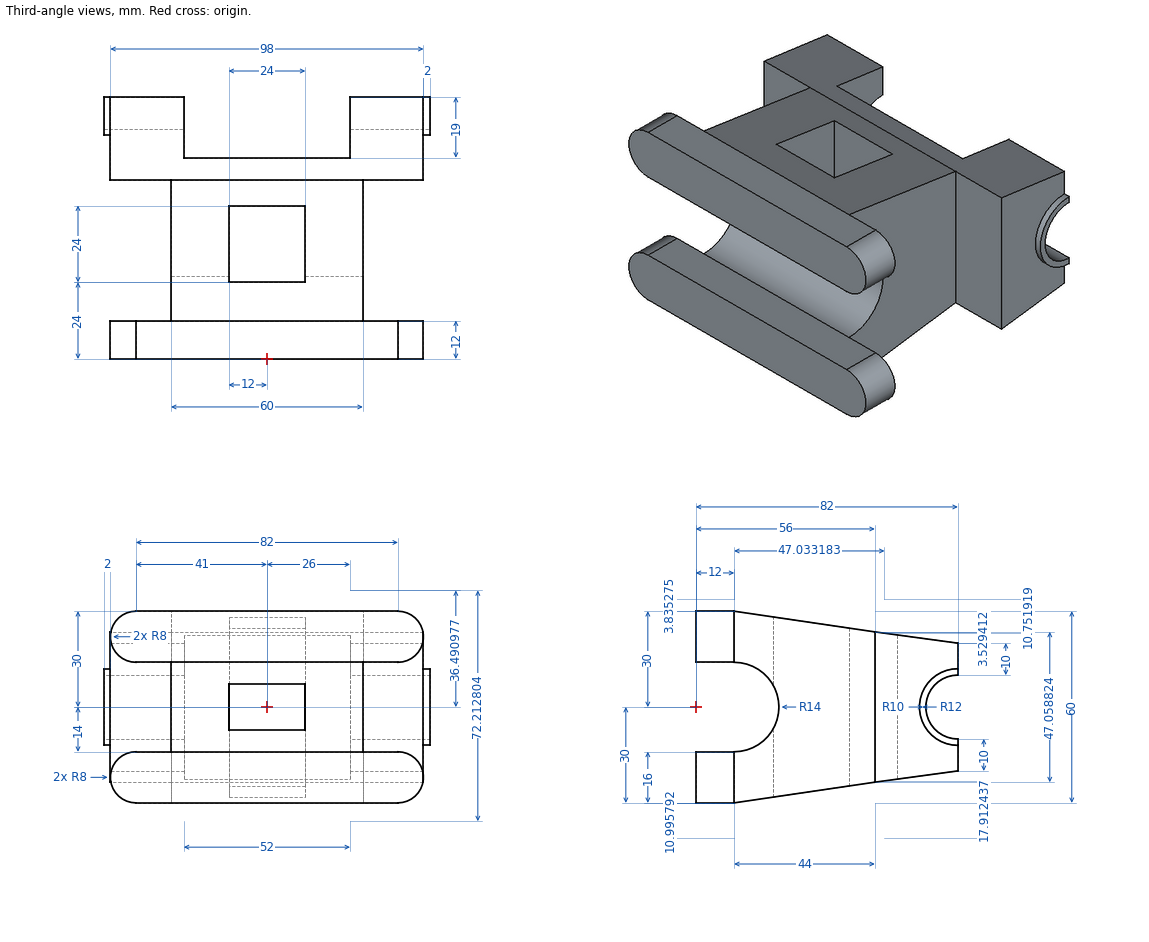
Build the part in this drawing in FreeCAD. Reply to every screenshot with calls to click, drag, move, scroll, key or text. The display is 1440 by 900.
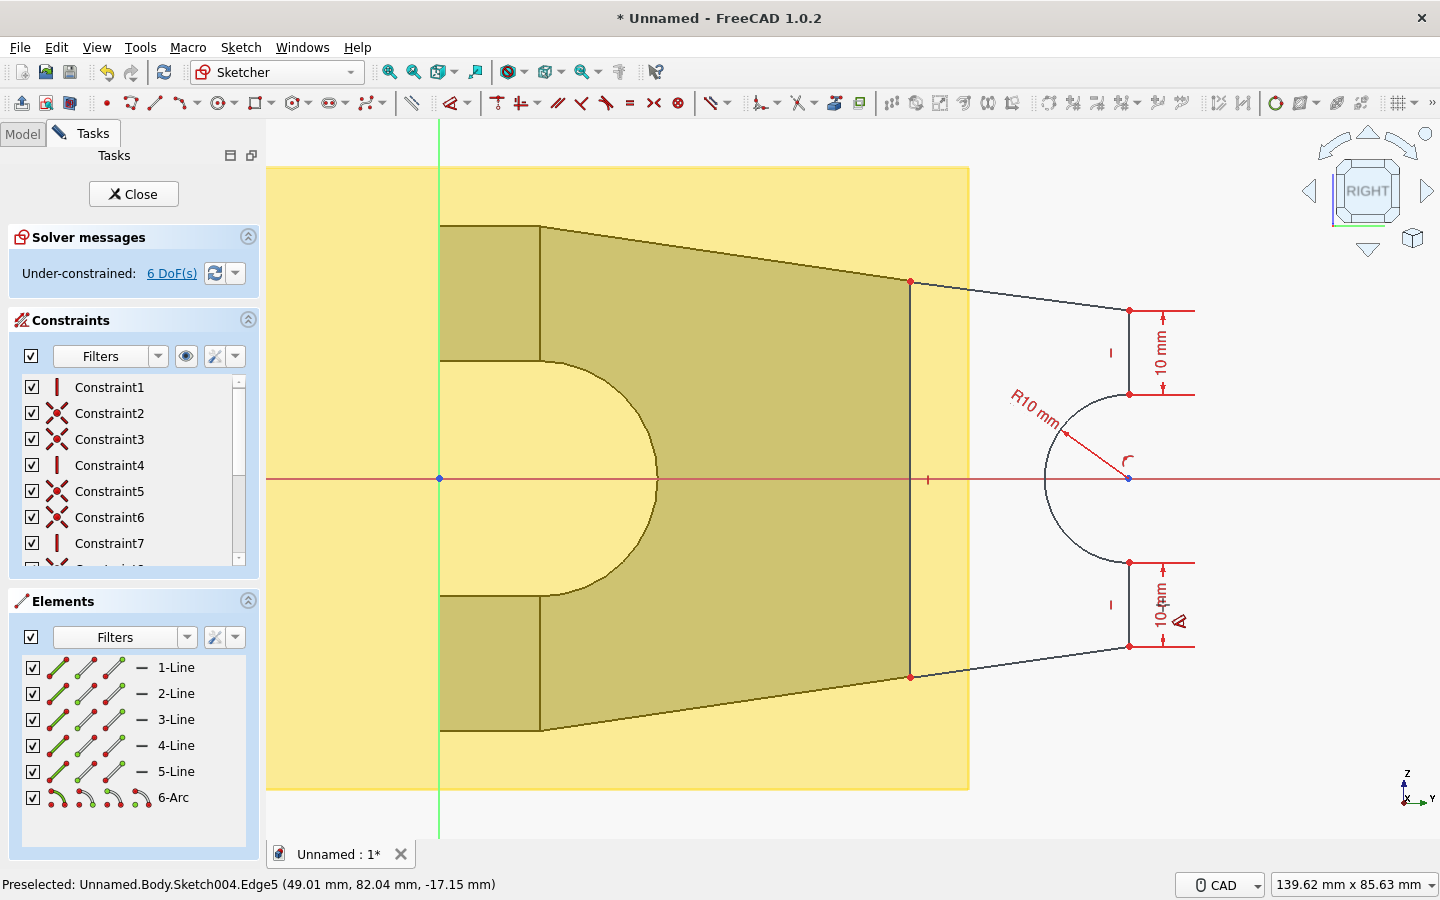
click(1129, 395)
click(784, 361)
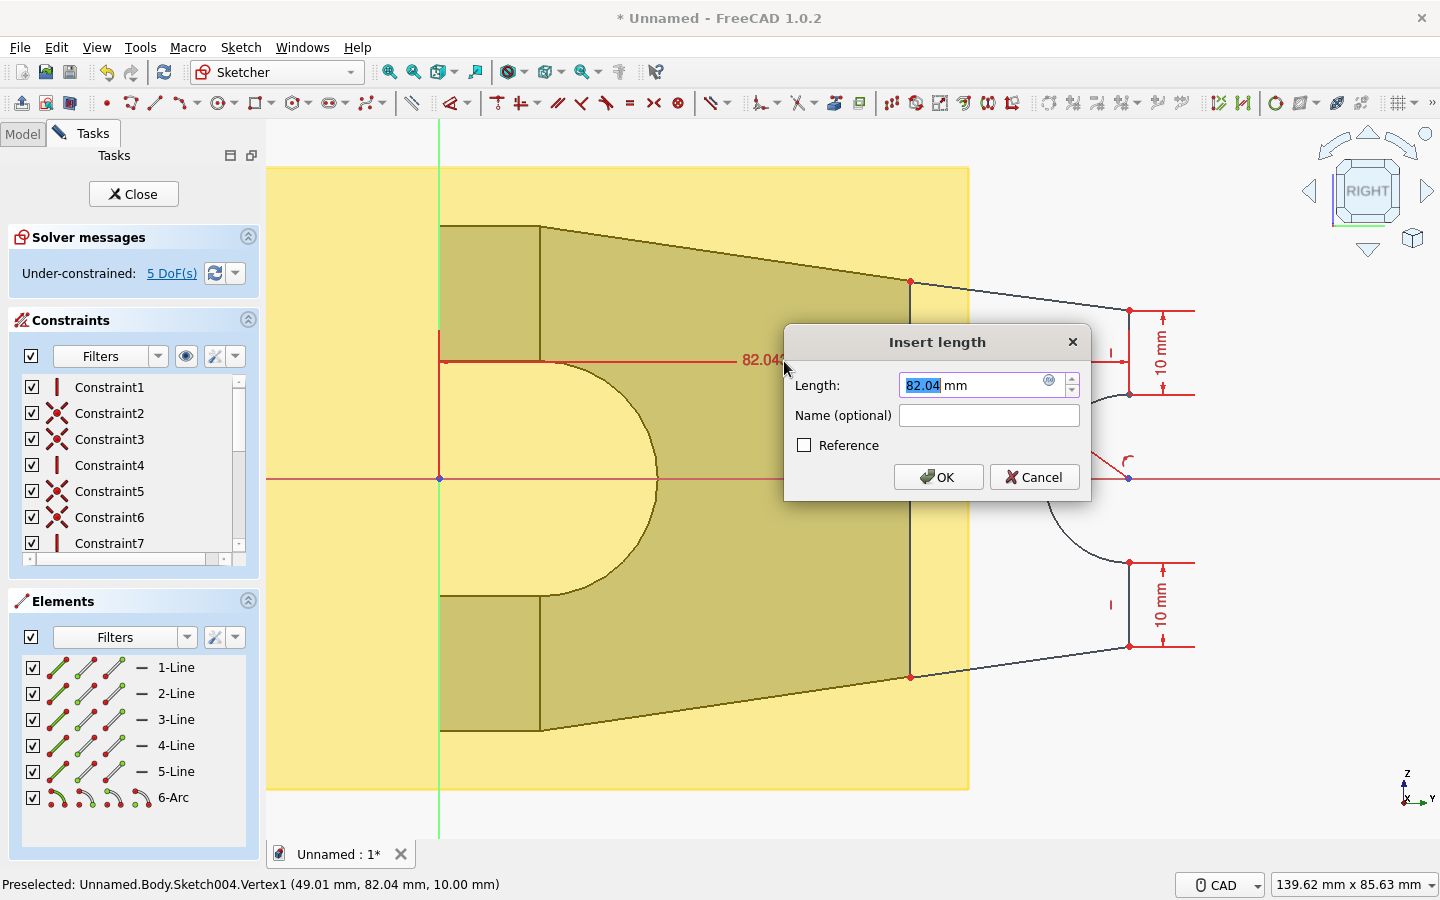
text(82)
key(Return)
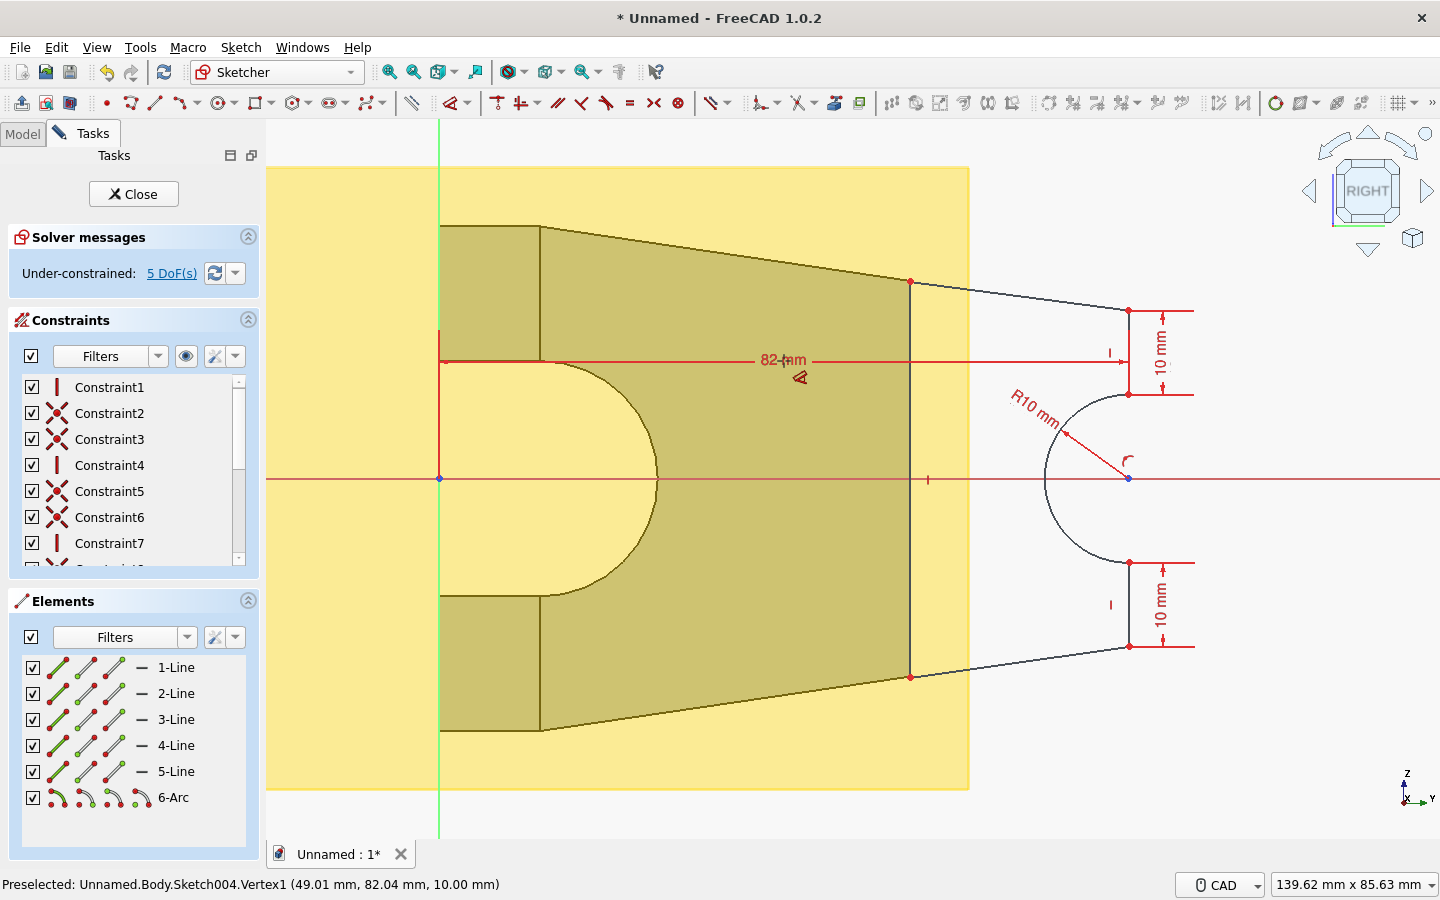
click(910, 282)
click(675, 248)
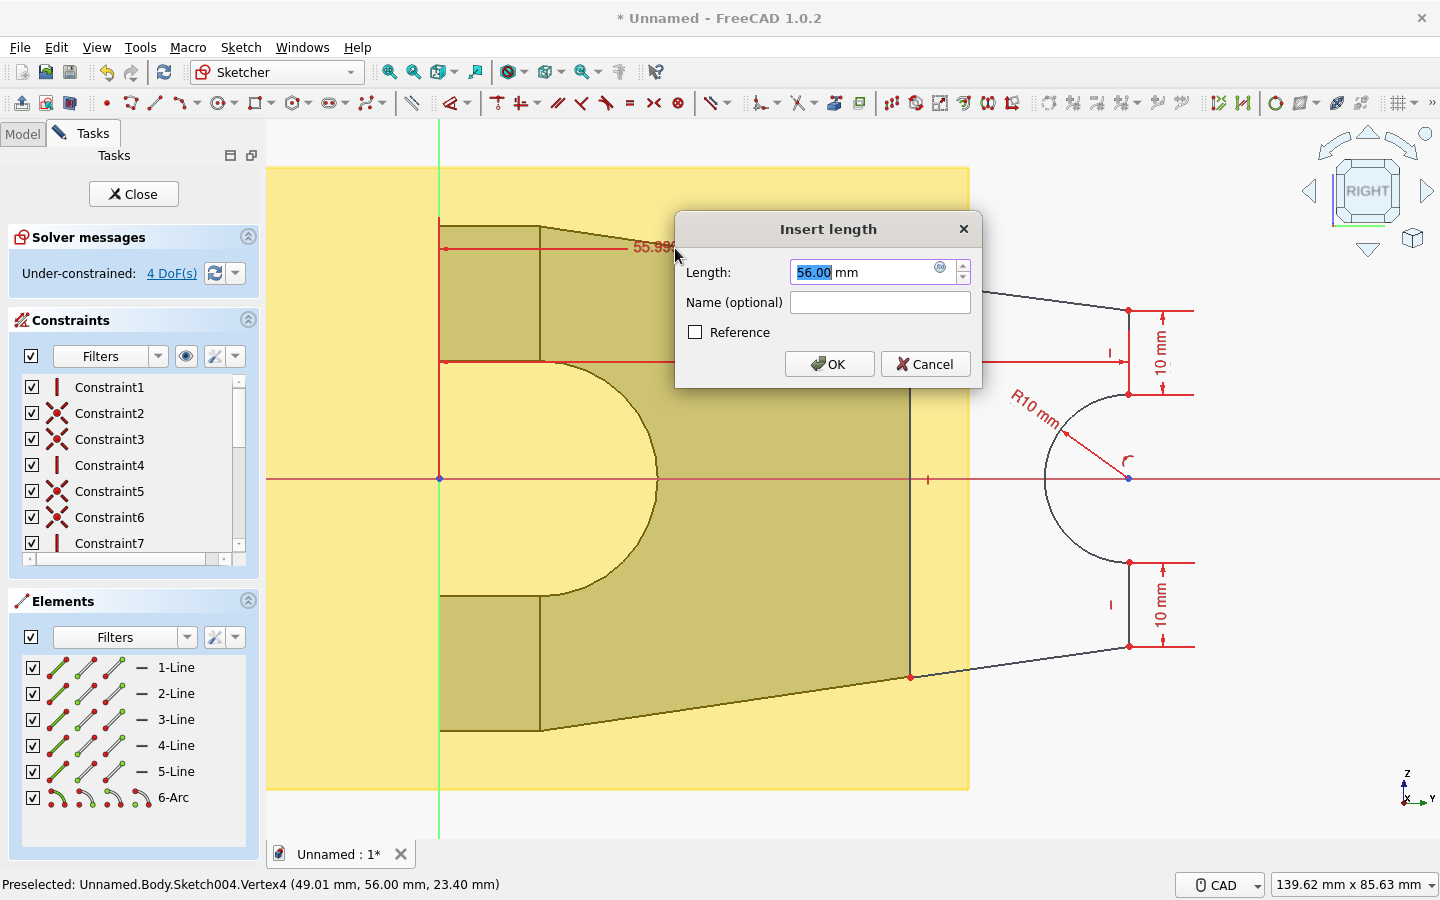
text(56)
key(Return)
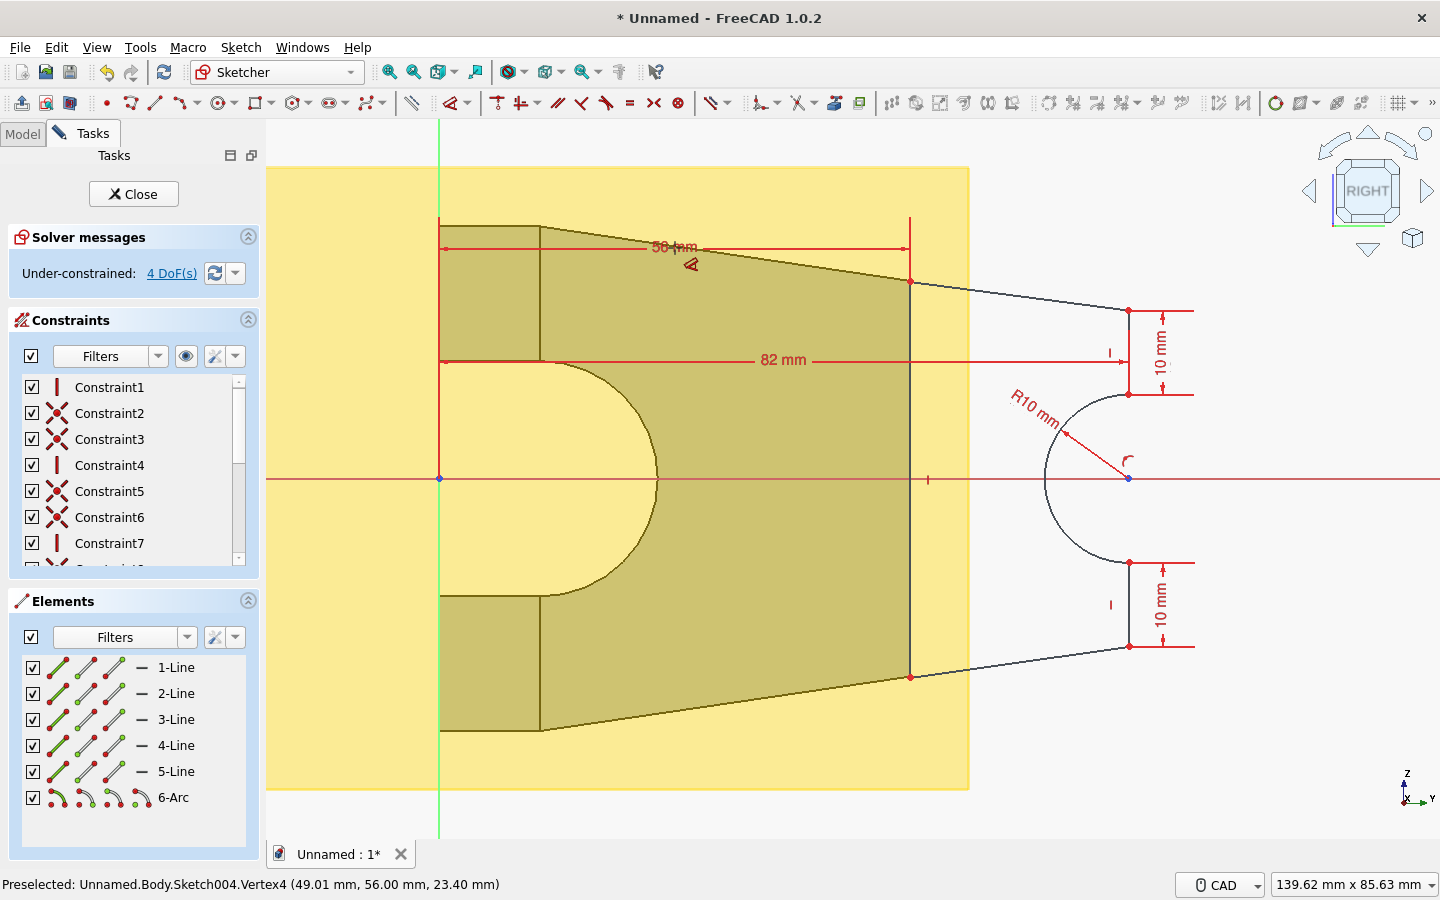
click(1129, 647)
click(784, 681)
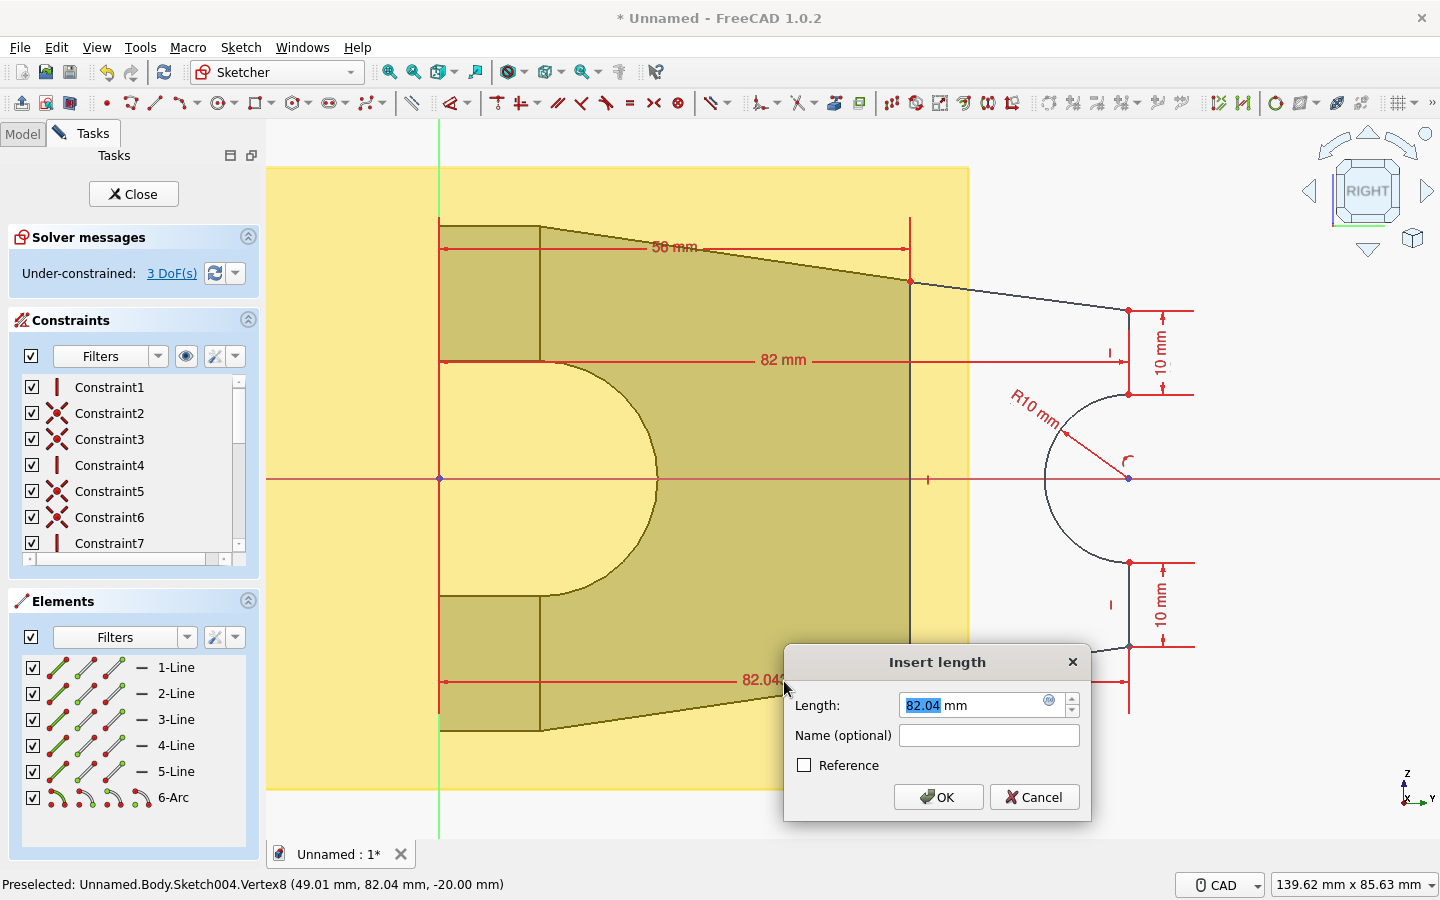
text(82)
key(Return)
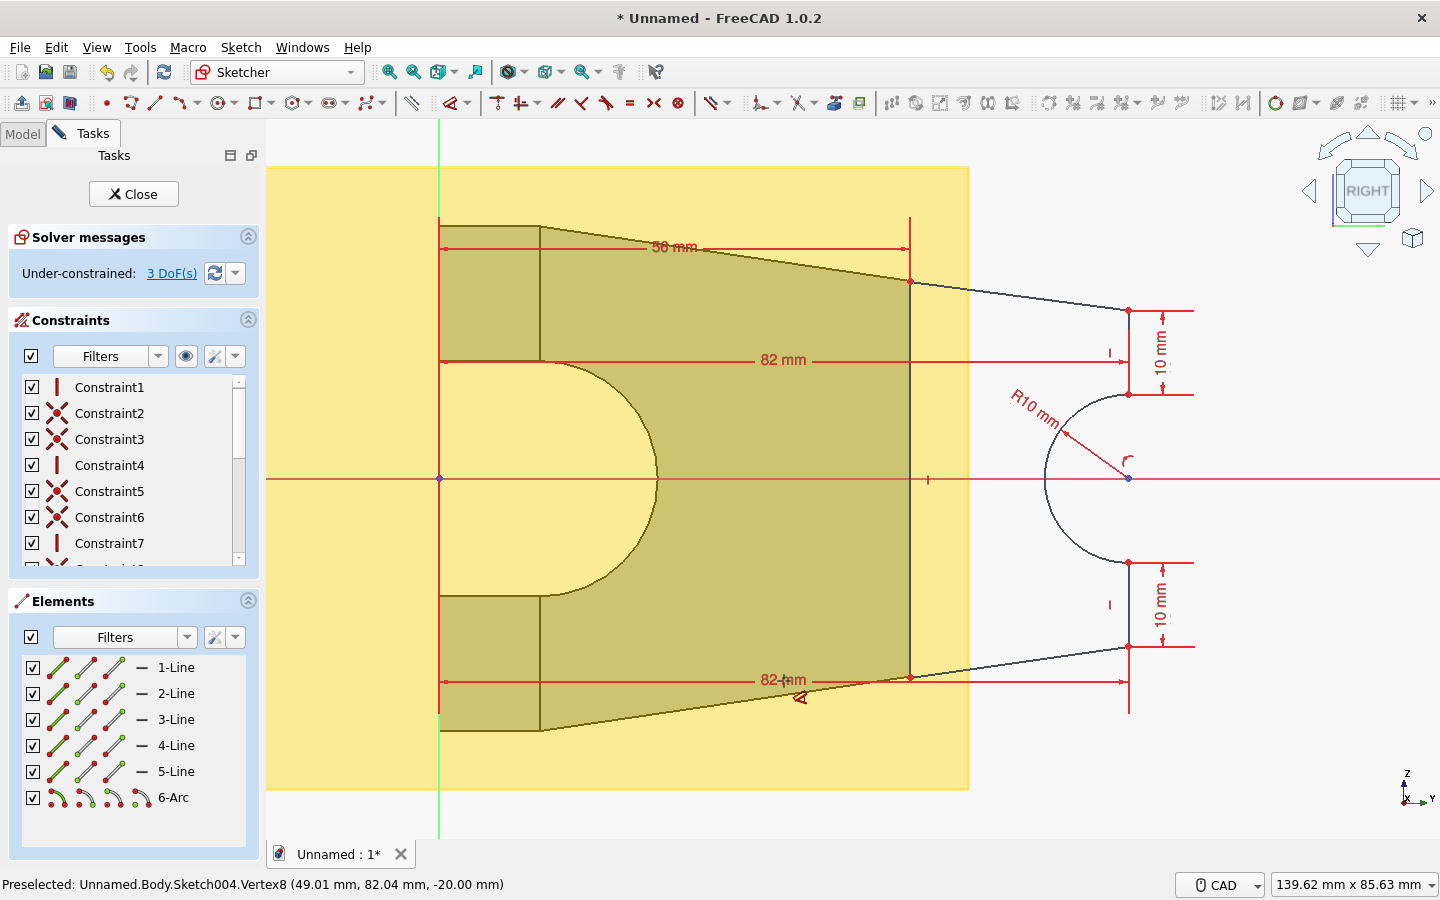
click(1129, 479)
click(784, 513)